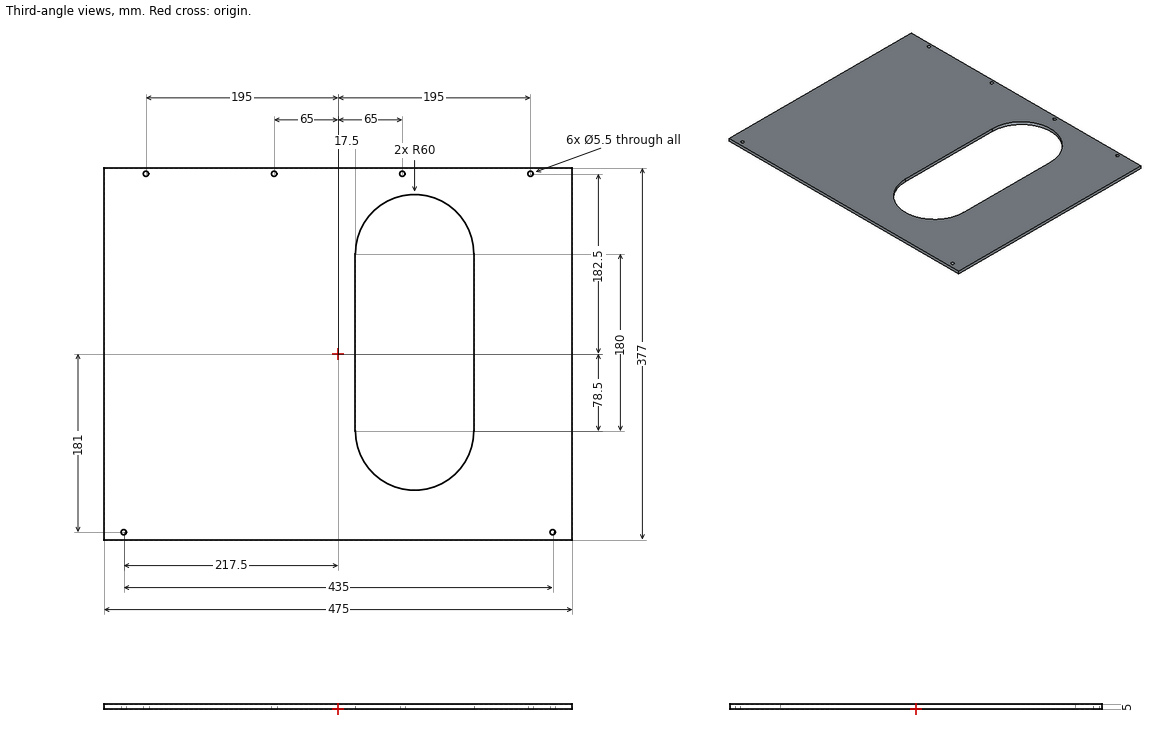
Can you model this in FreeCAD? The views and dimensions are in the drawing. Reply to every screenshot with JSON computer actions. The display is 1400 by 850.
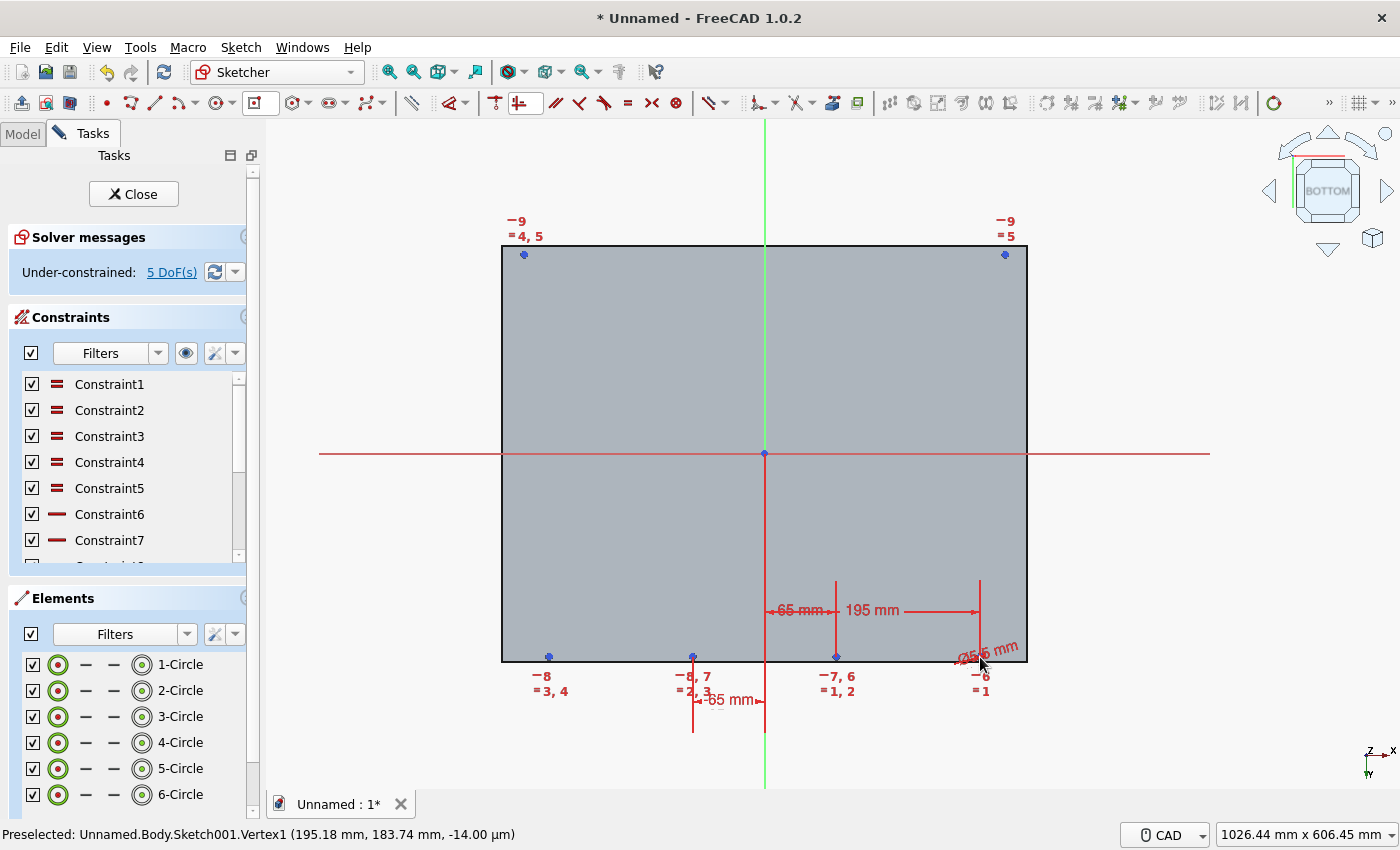
{"action": "left_click", "coordinate": [549, 657]}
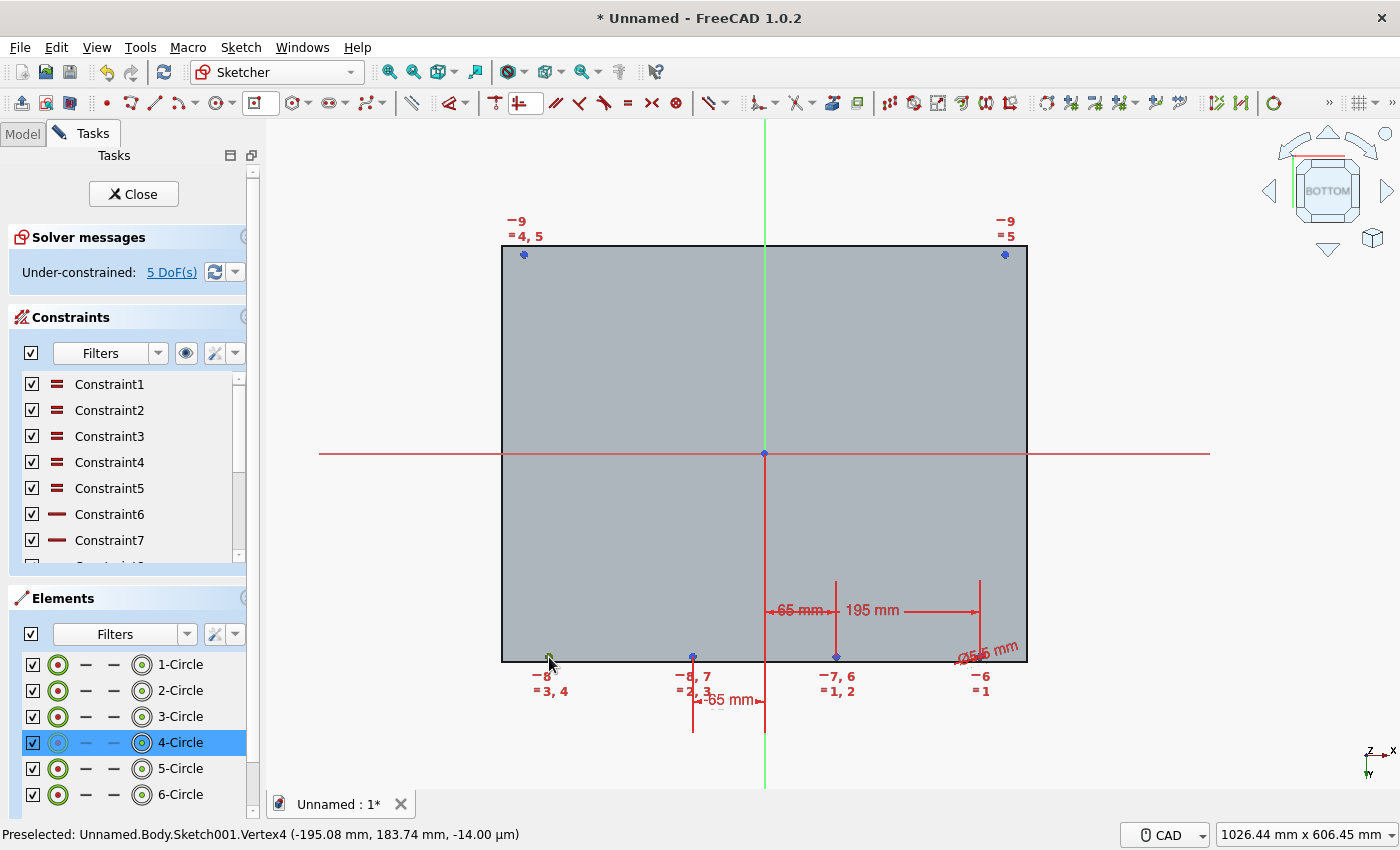
{"action": "key", "text": "l"}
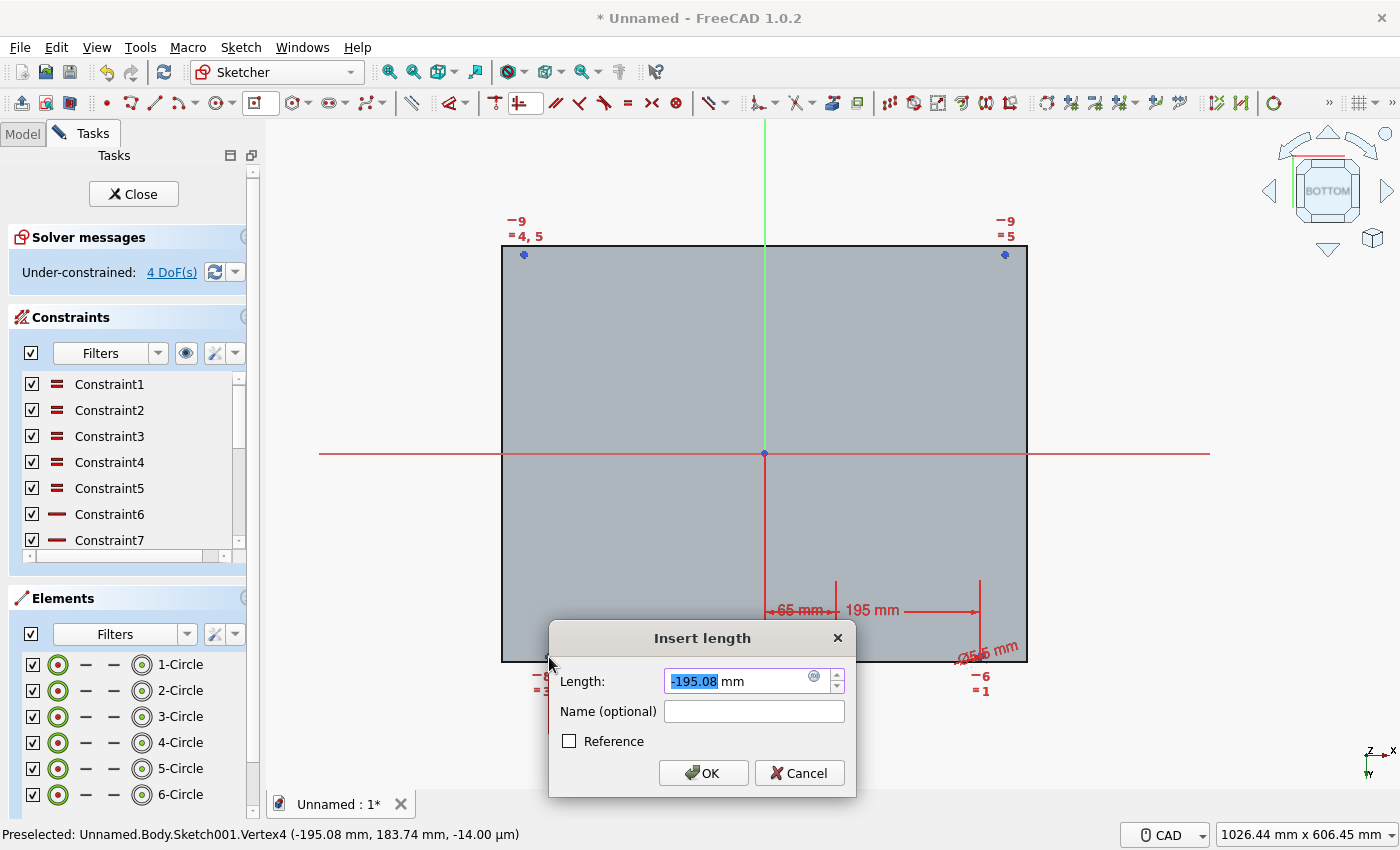
{"action": "type", "text": "-195"}
{"action": "key", "text": "Return"}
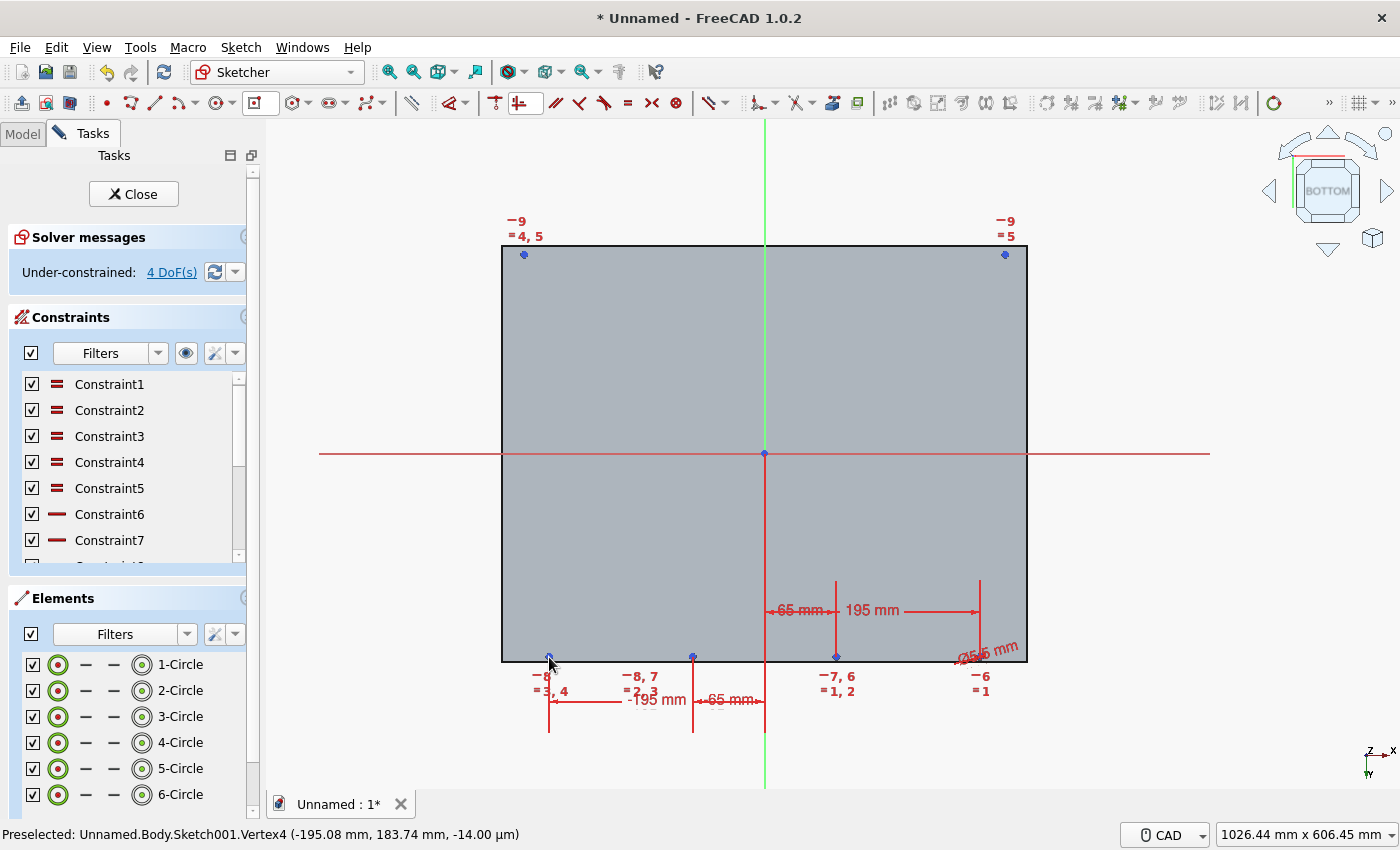
{"action": "left_click", "coordinate": [524, 255]}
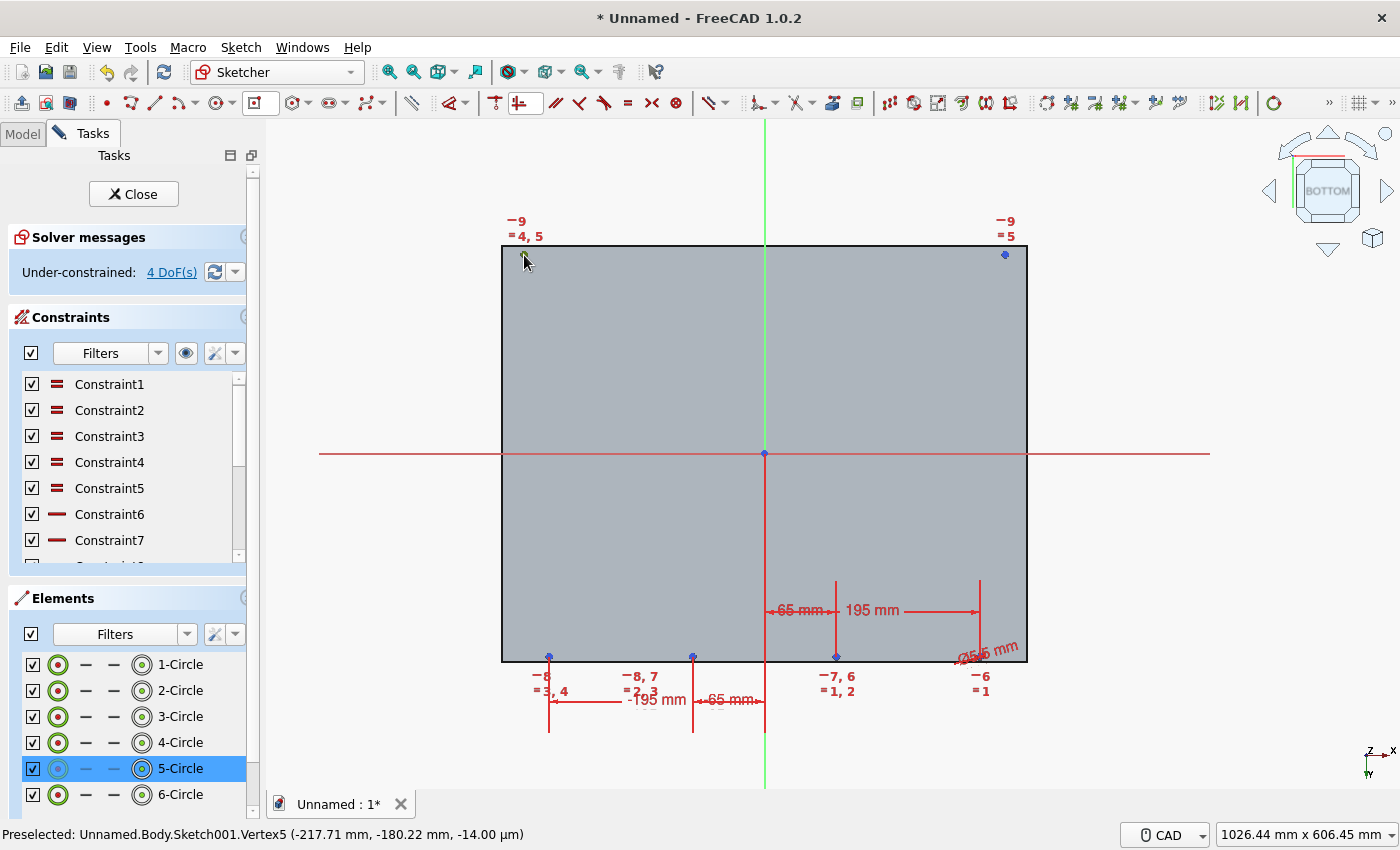
{"action": "key", "text": "i"}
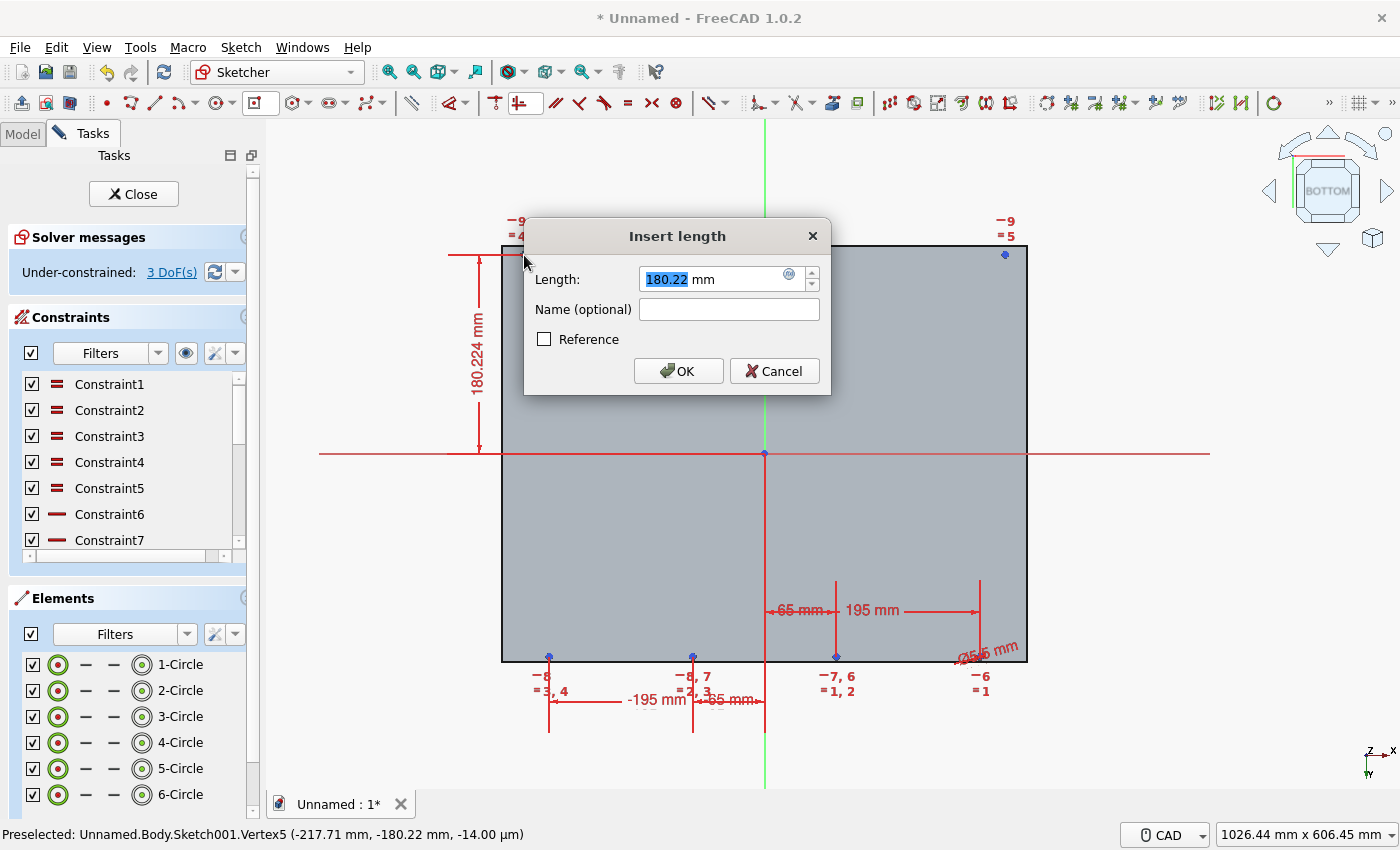
{"action": "type", "text": "181"}
{"action": "key", "text": "Return"}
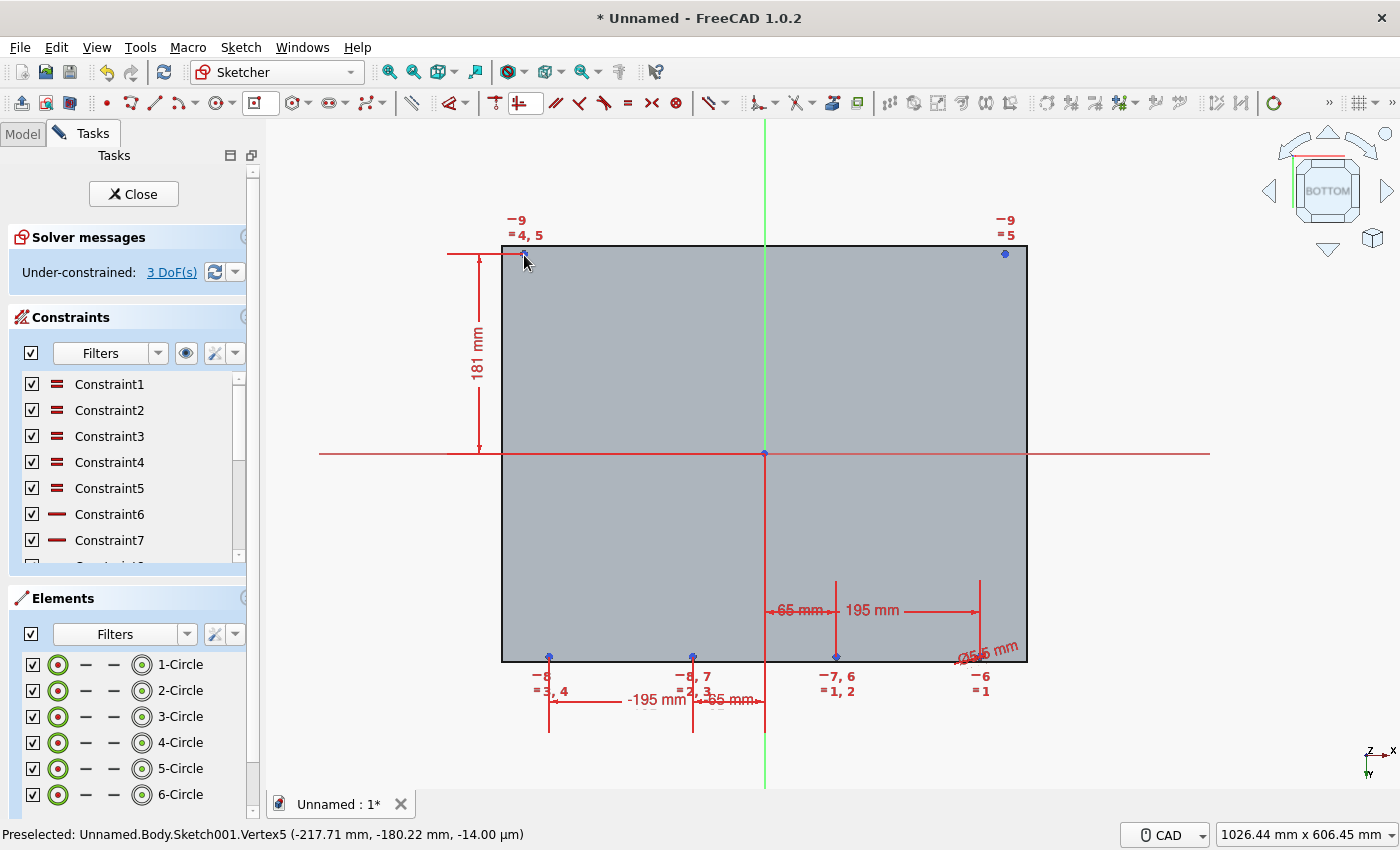
{"action": "left_click", "coordinate": [524, 254]}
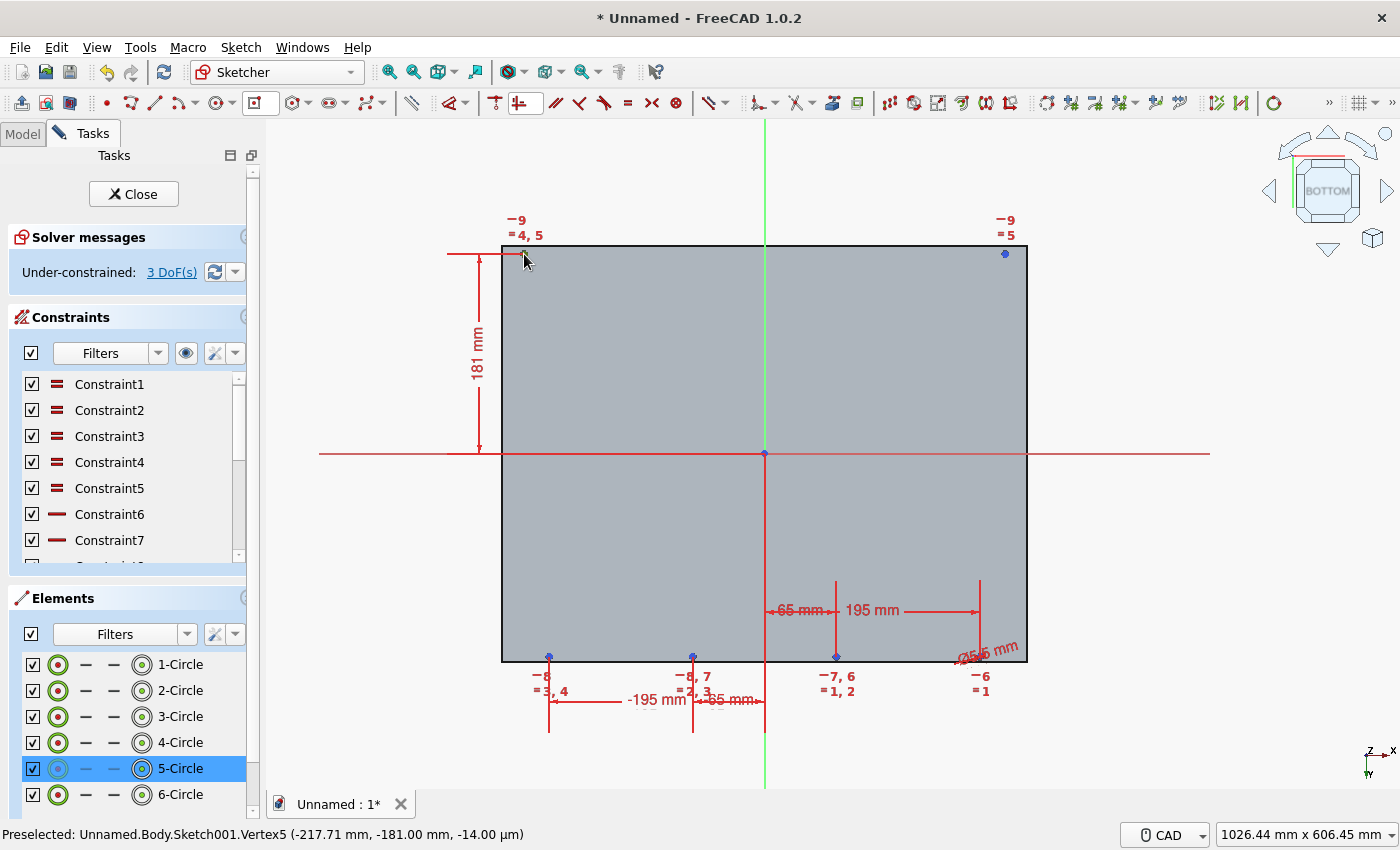
{"action": "left_click", "coordinate": [1005, 254]}